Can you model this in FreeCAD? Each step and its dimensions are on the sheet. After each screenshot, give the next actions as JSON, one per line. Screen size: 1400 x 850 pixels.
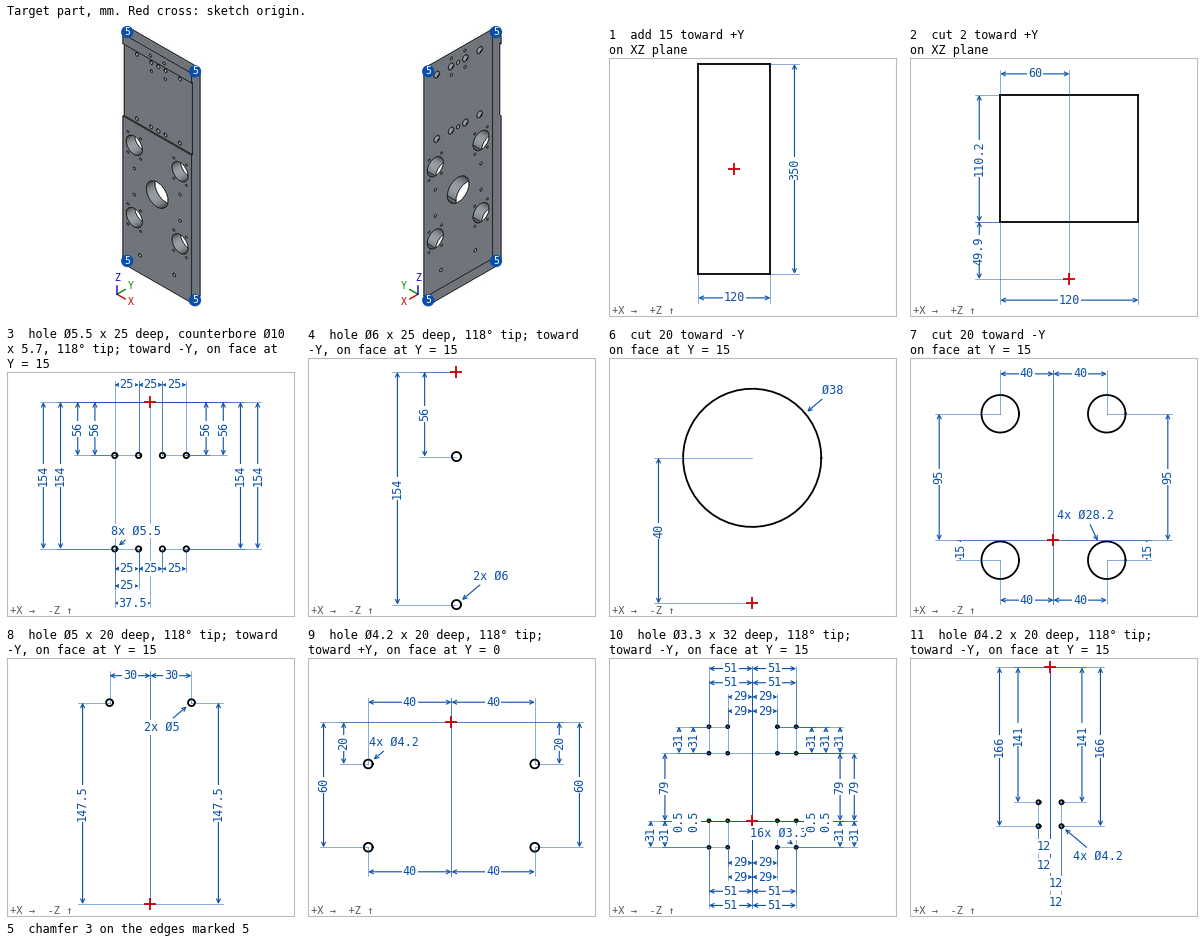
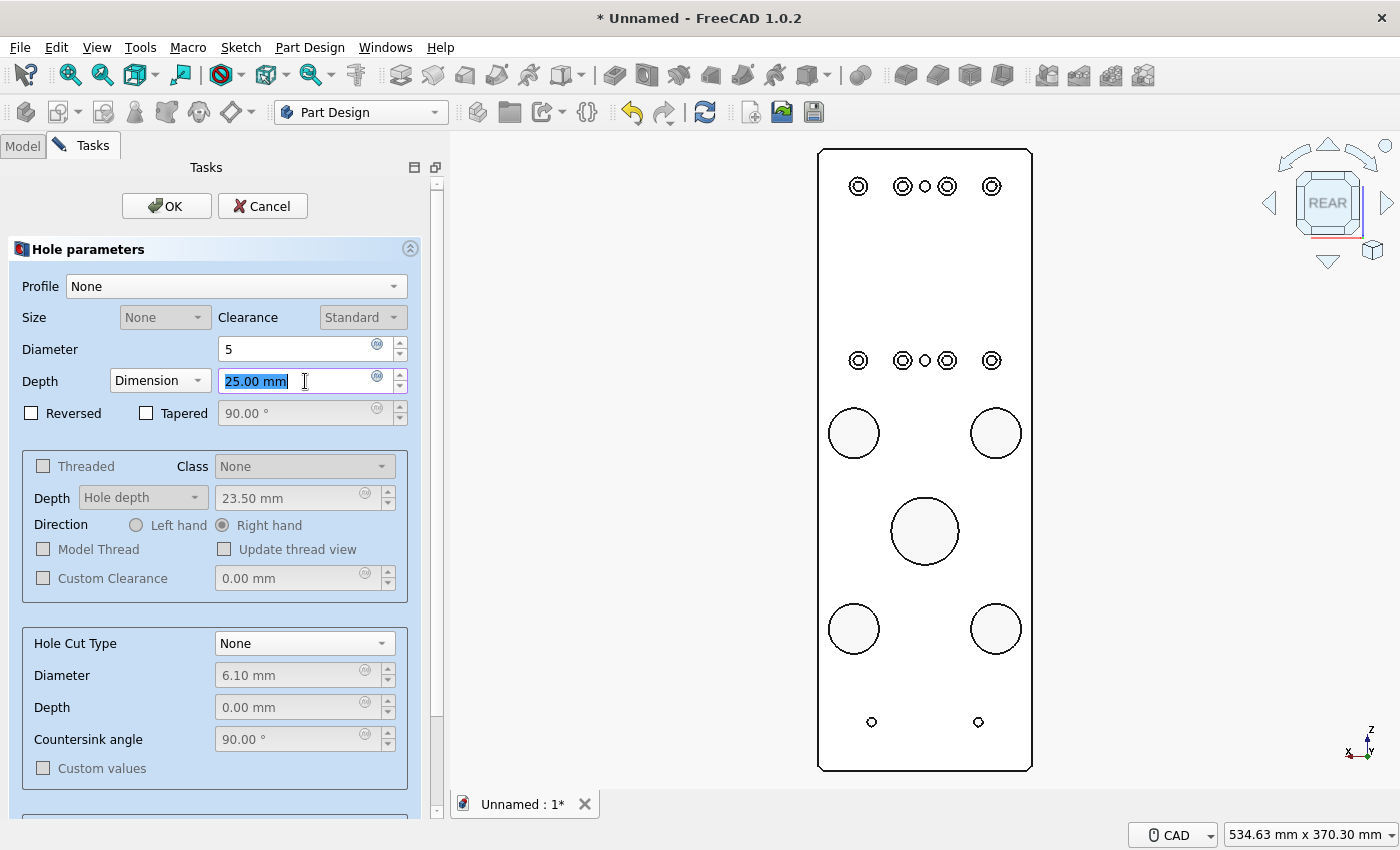
{"action": "type", "text": "20"}
{"action": "key", "text": "Tab"}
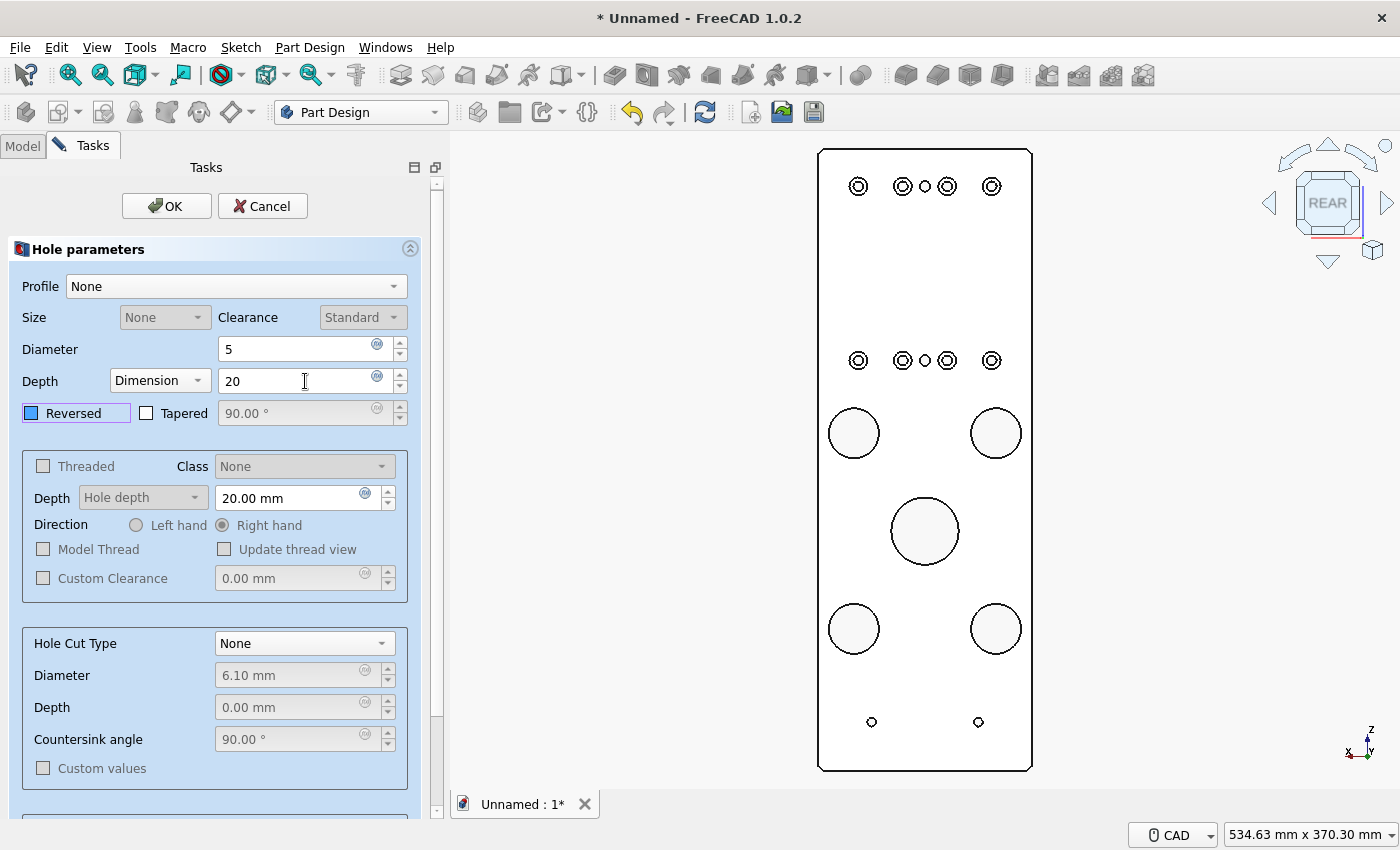
{"action": "left_click", "coordinate": [167, 206]}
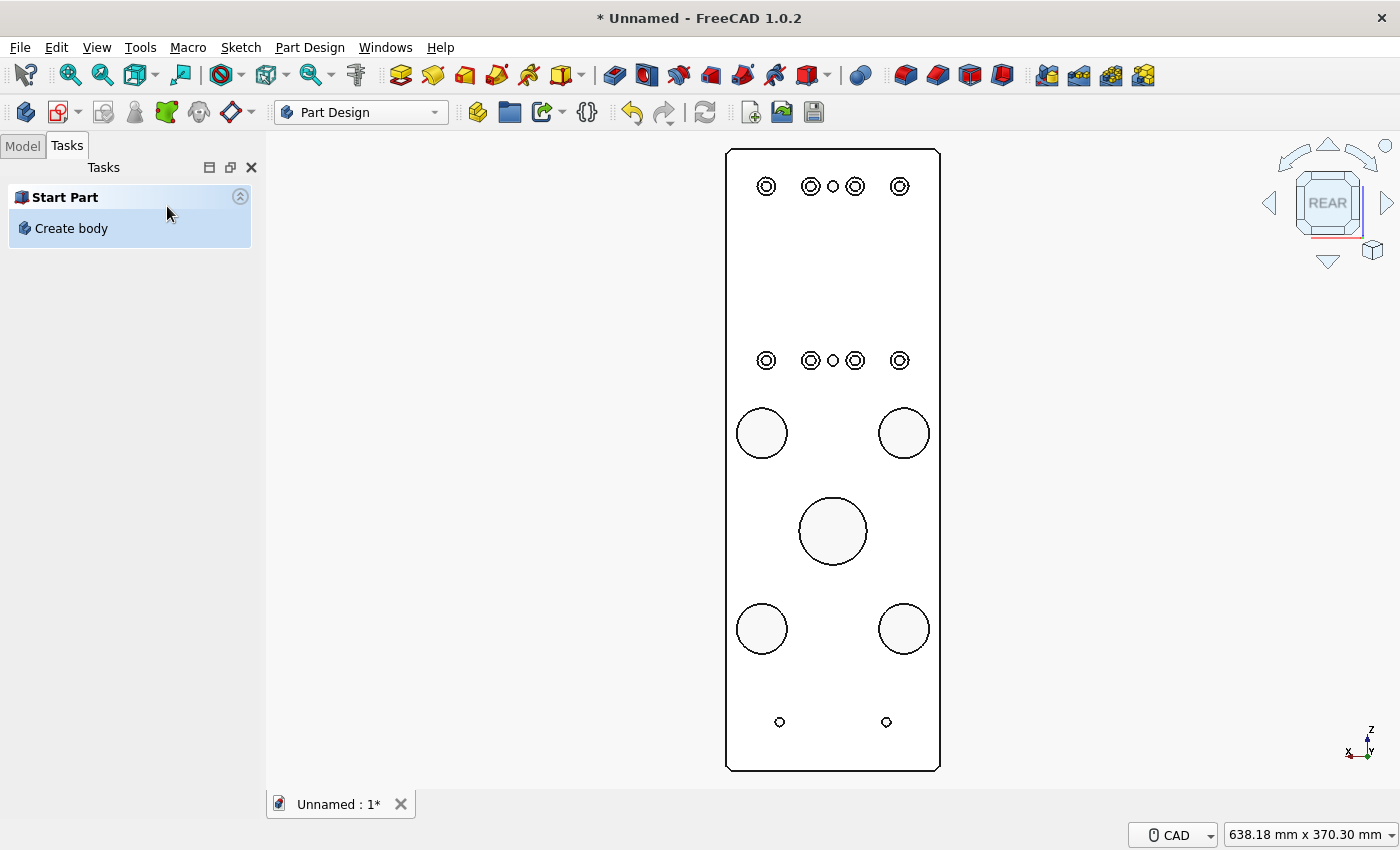
{"action": "key", "text": "0"}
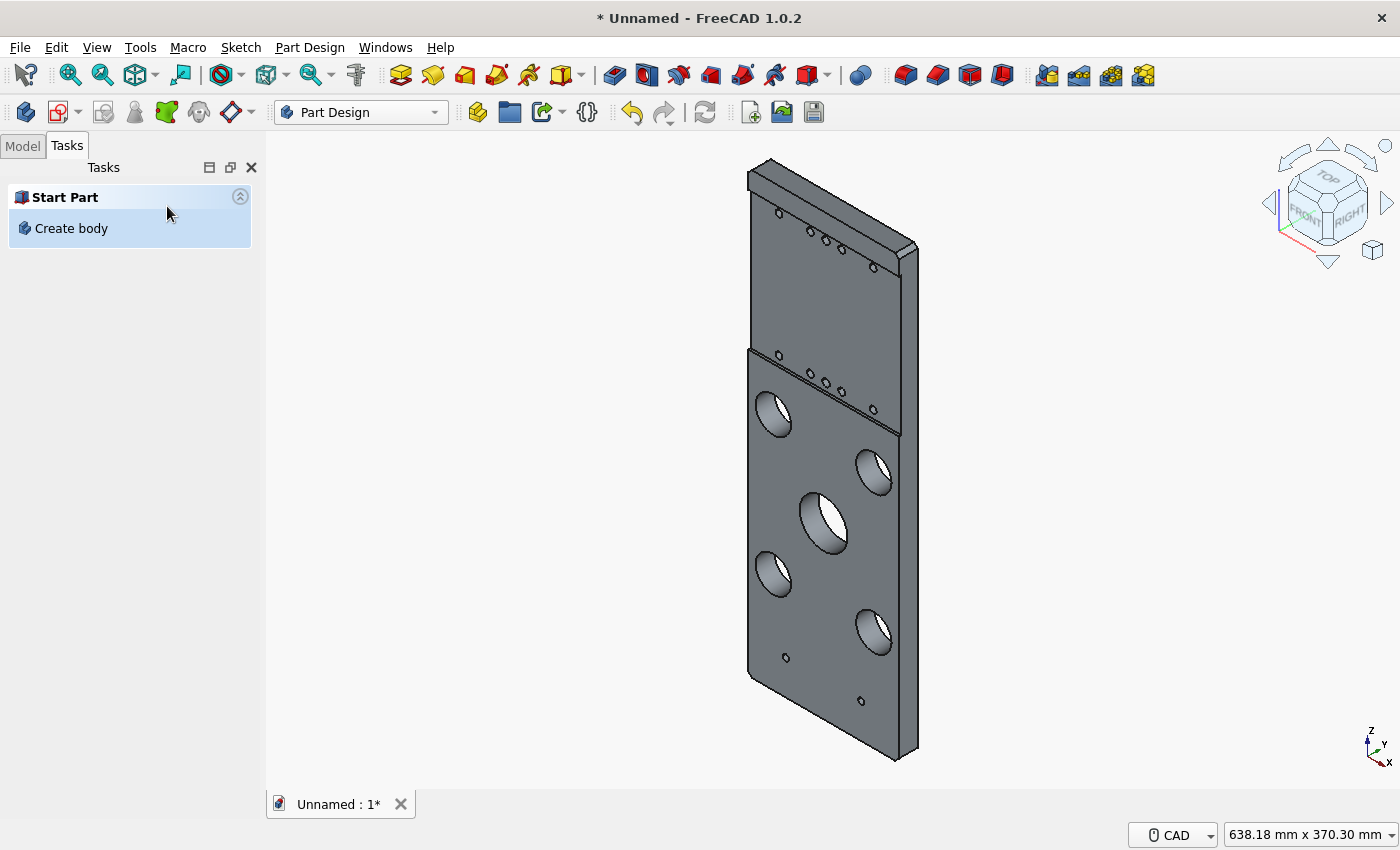
{"action": "left_click", "coordinate": [824, 648]}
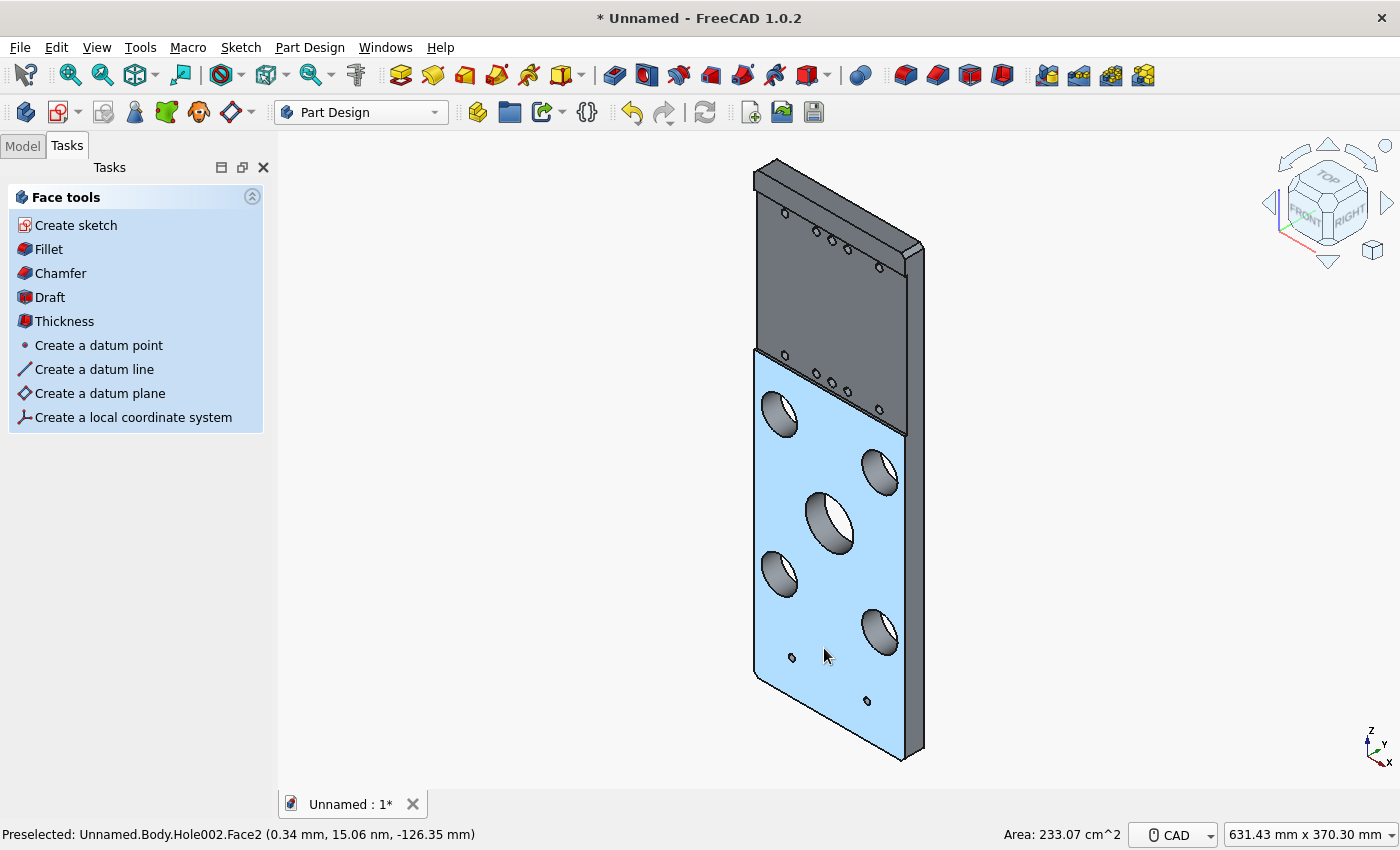
{"action": "left_click", "coordinate": [58, 112]}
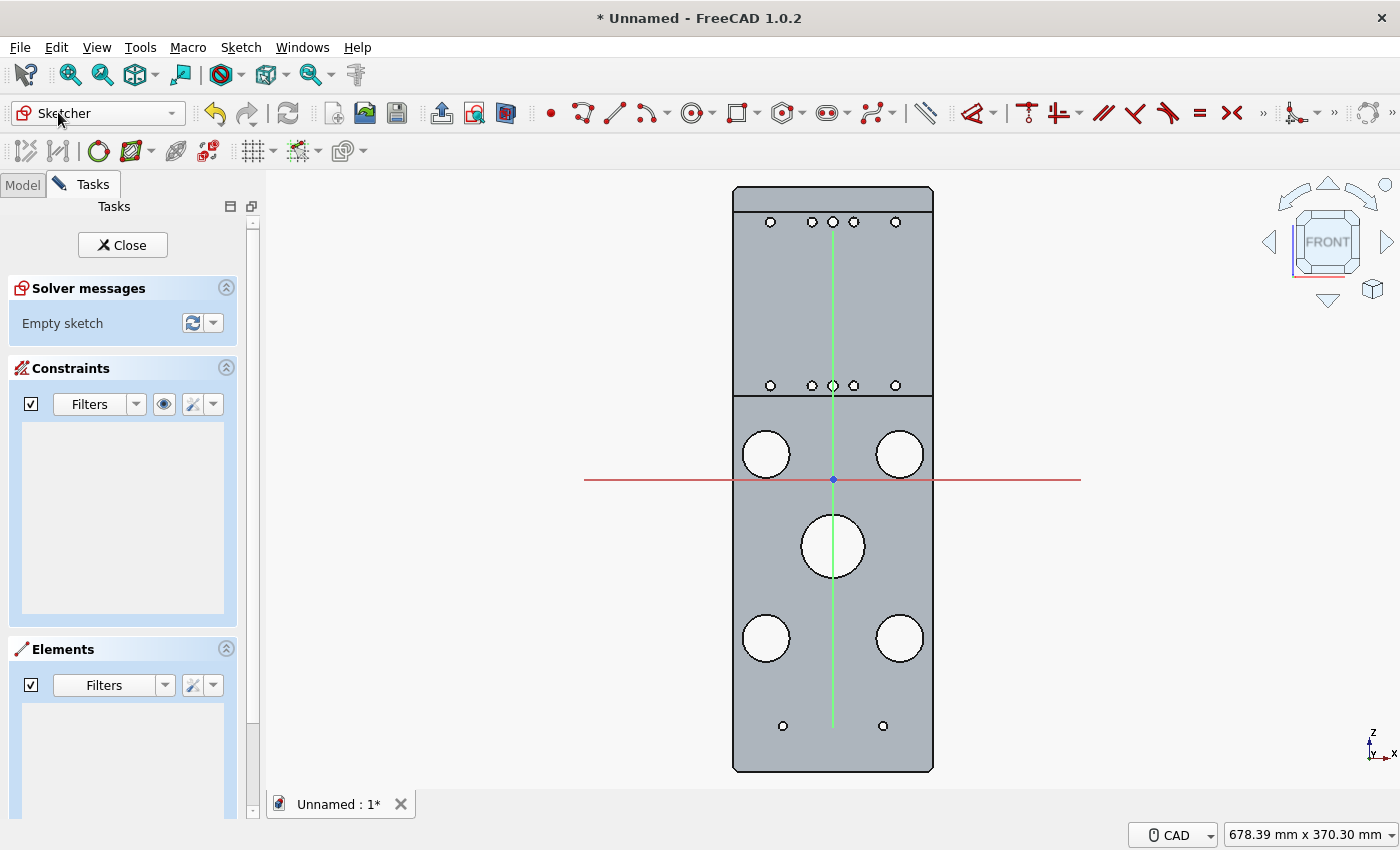
{"action": "scroll", "coordinate": [855, 548], "scroll_direction": "up", "scroll_amount": 7}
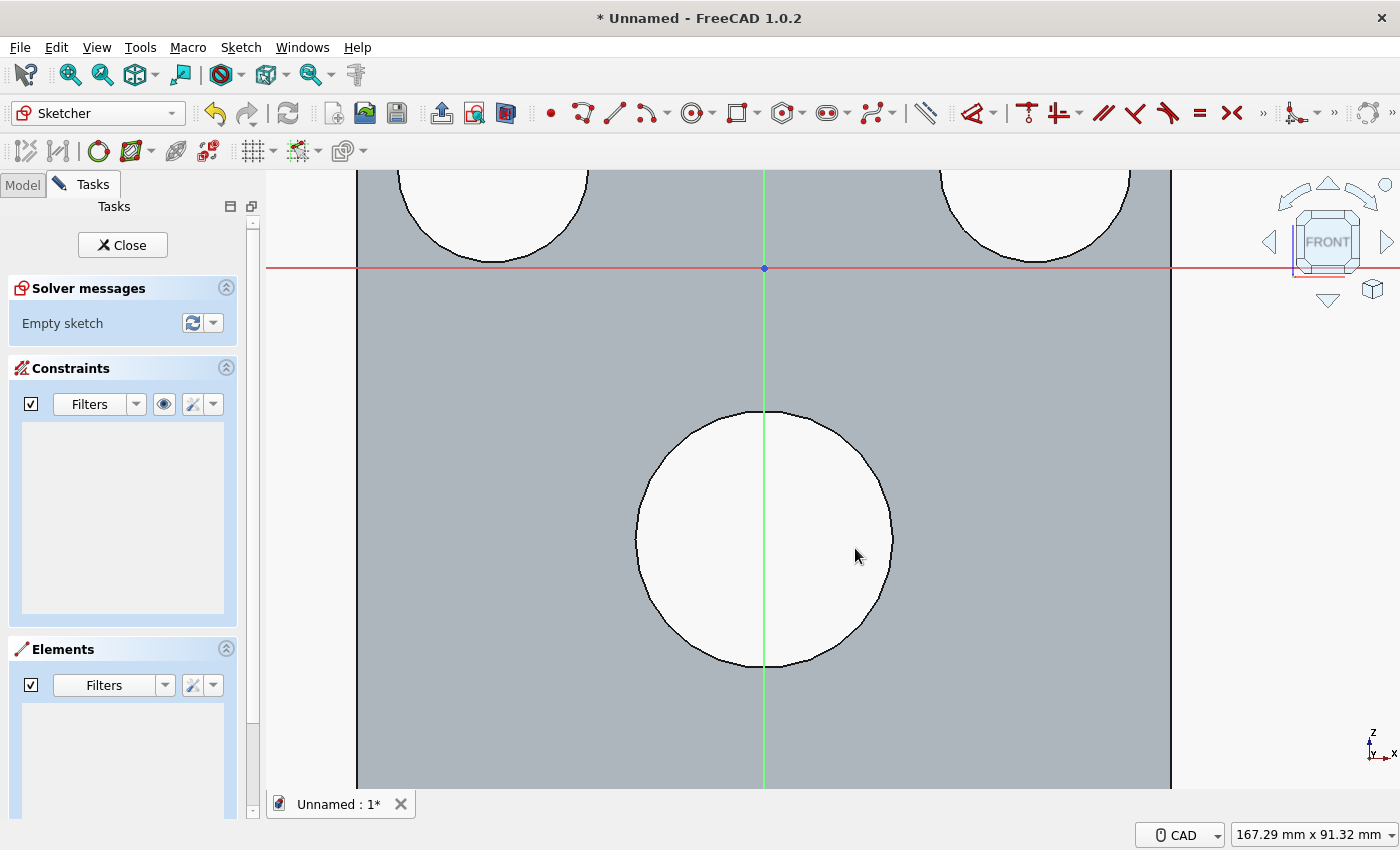
{"action": "left_click", "coordinate": [692, 114]}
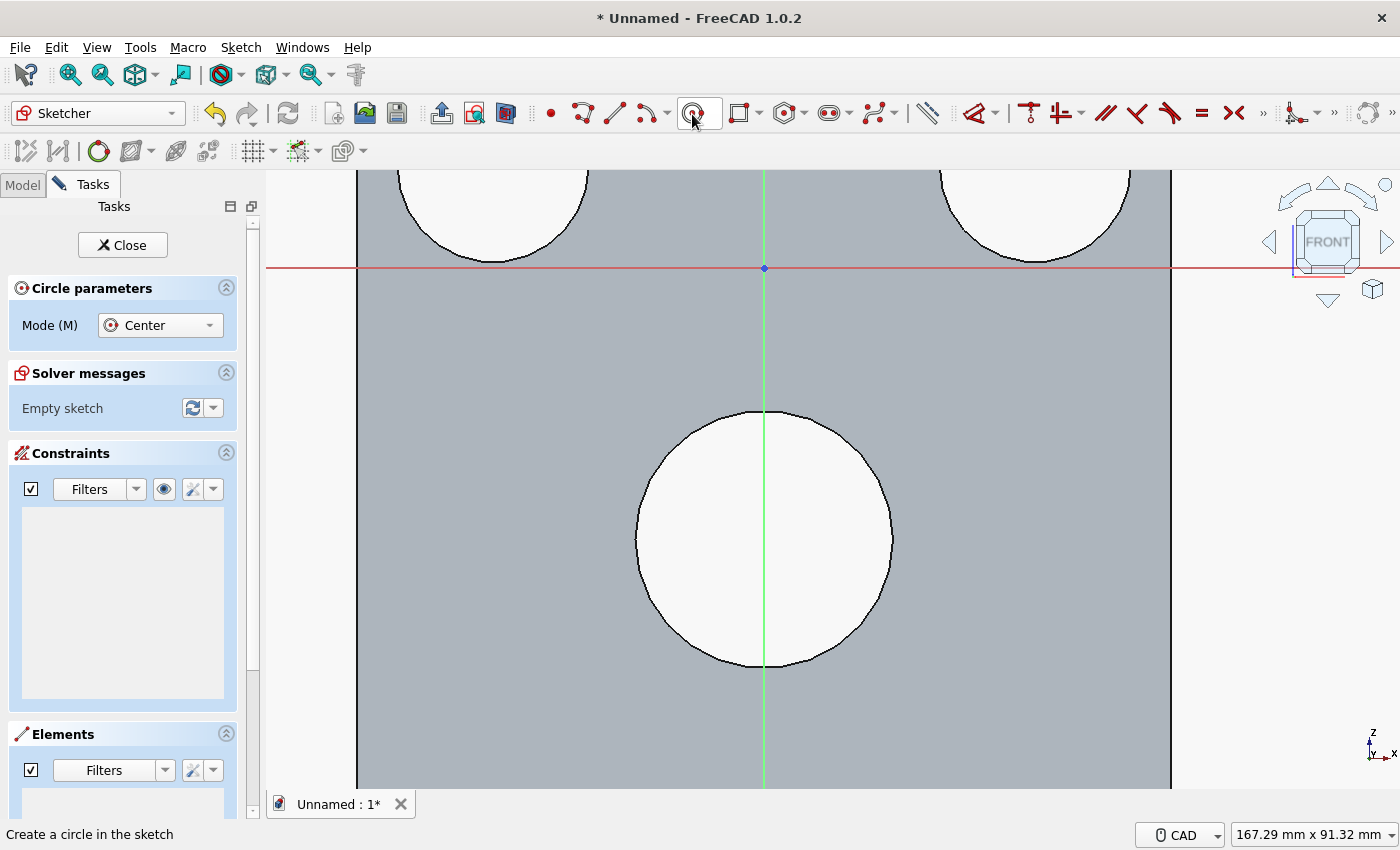
{"action": "scroll", "coordinate": [493, 404], "scroll_direction": "up", "scroll_amount": 3}